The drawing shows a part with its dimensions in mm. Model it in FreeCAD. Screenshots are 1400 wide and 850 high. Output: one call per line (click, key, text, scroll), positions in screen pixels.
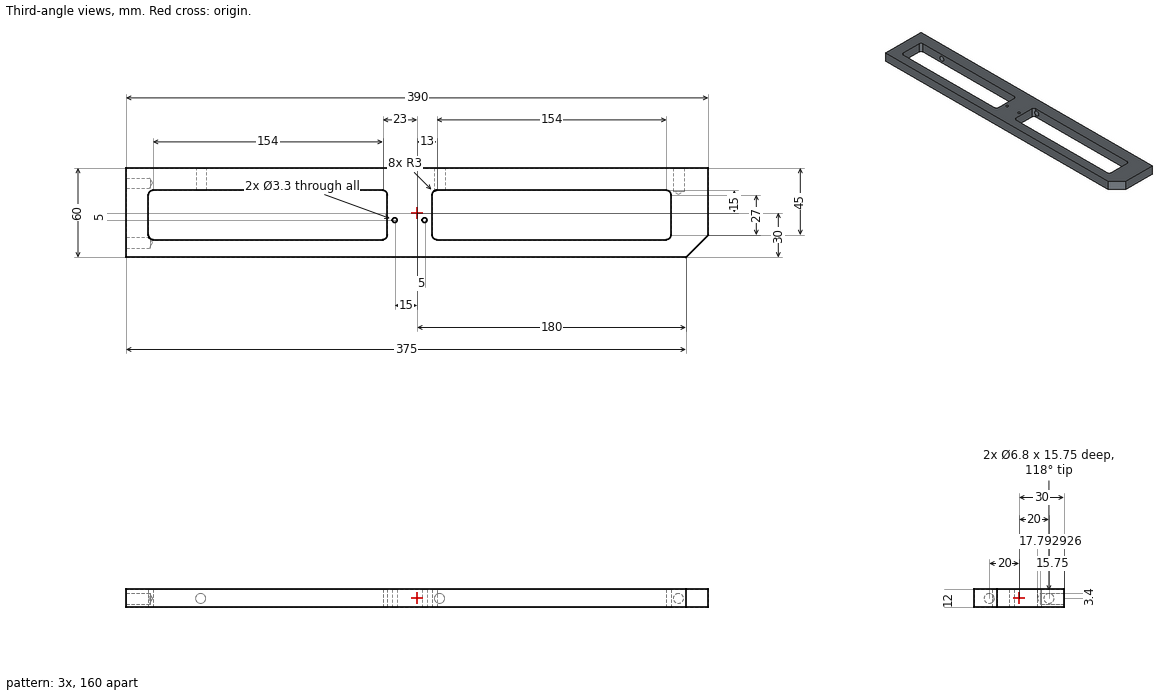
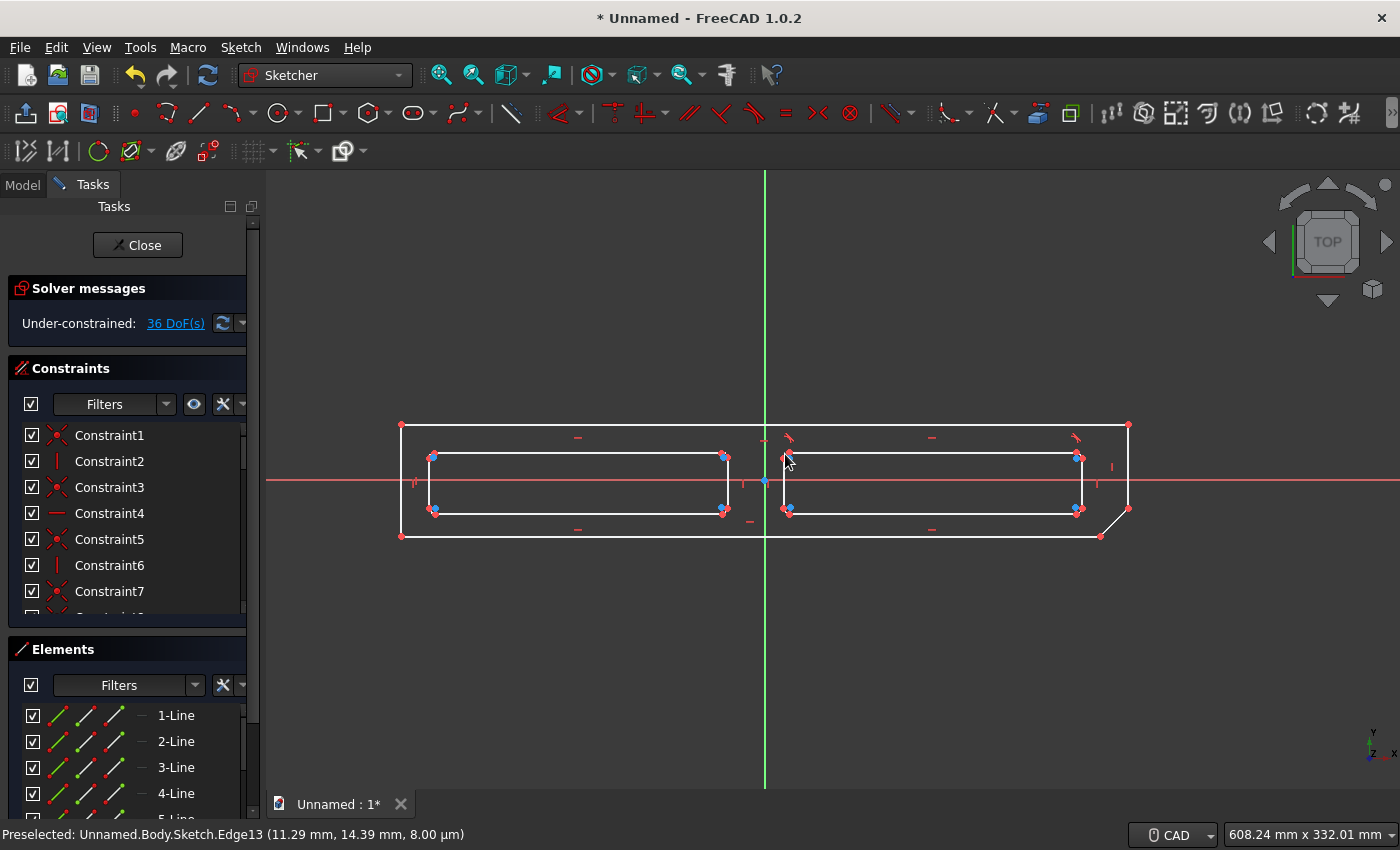
scroll(1082, 473, up, 4)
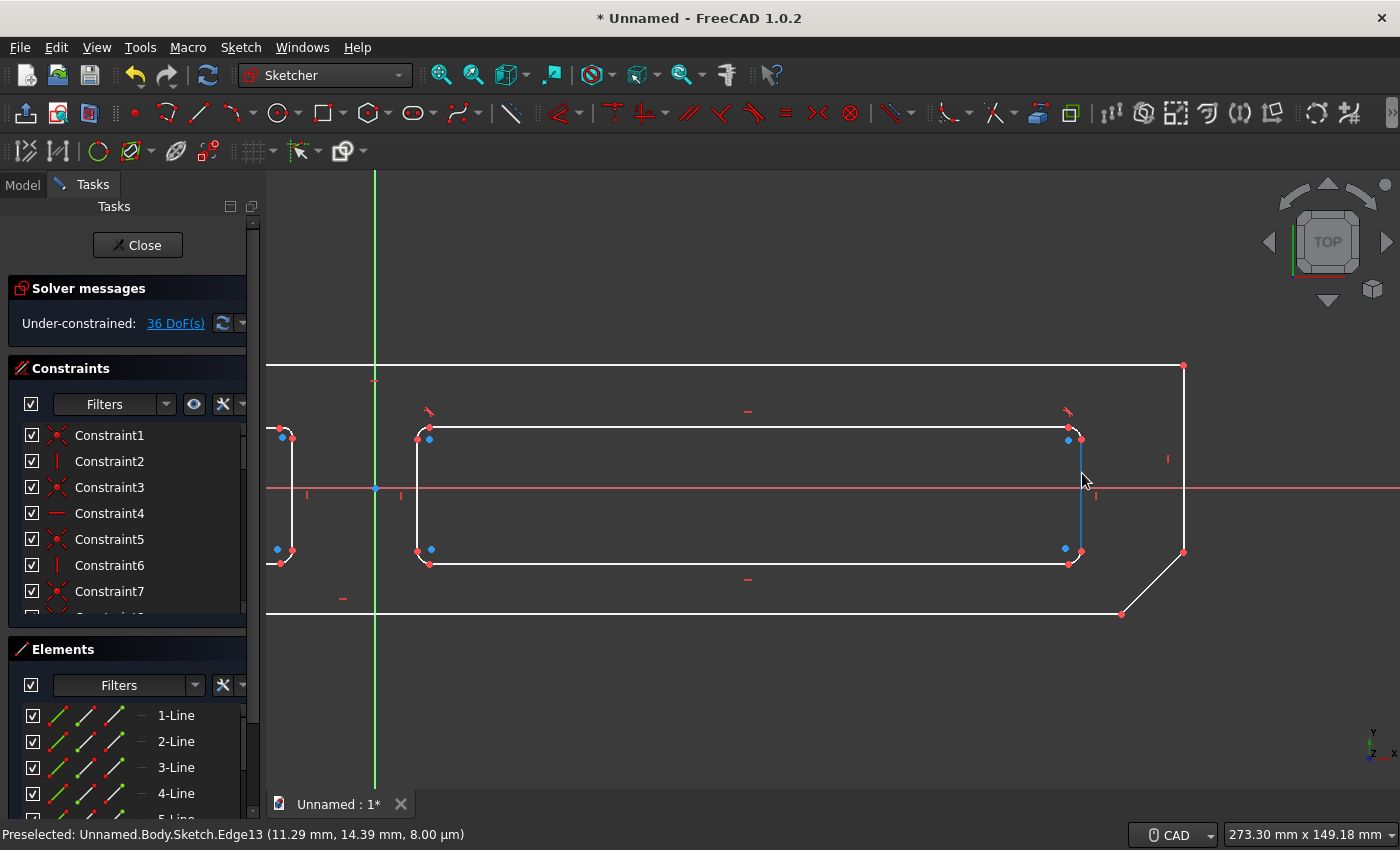
click(1081, 473)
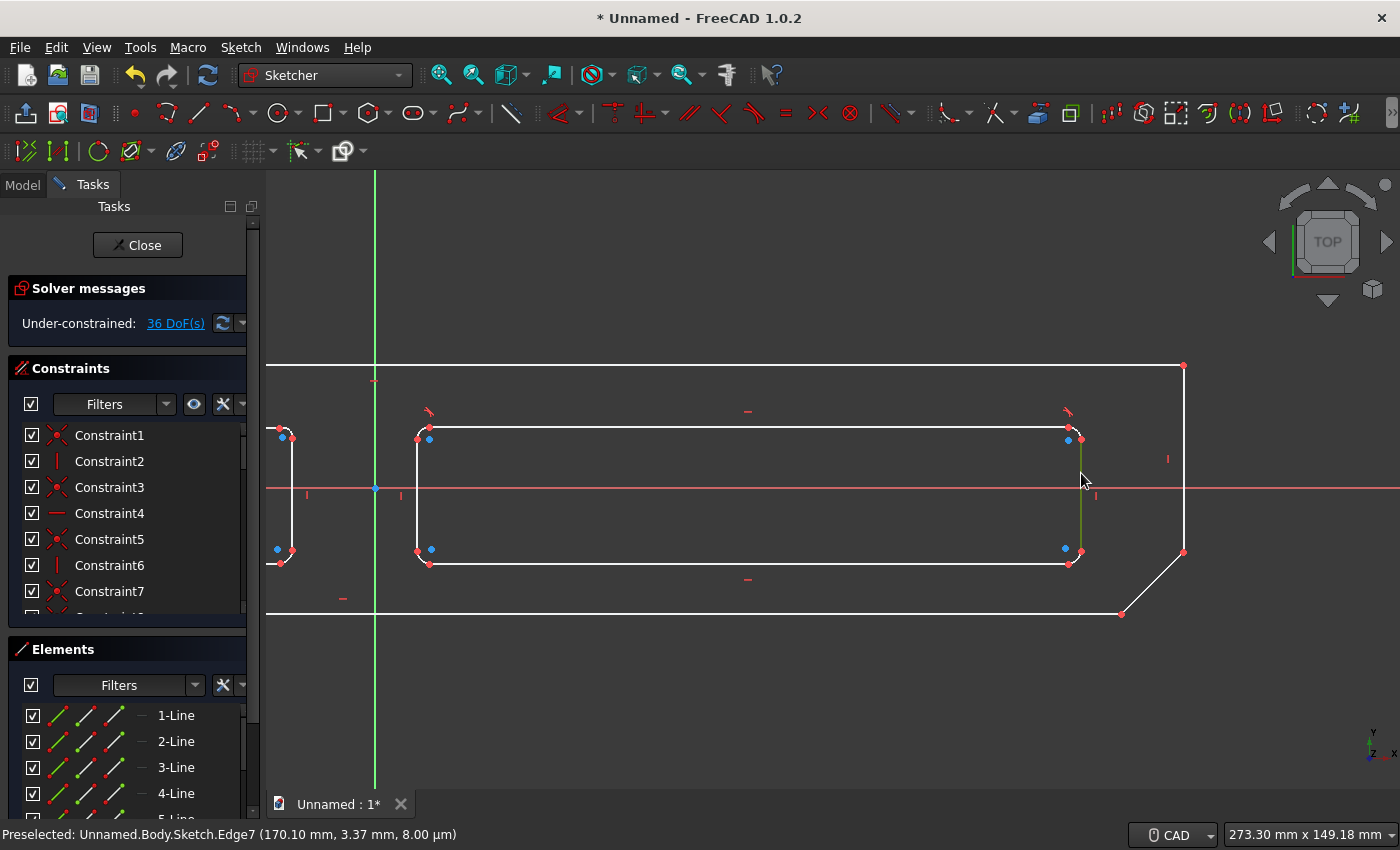
scroll(1077, 431, up, 2)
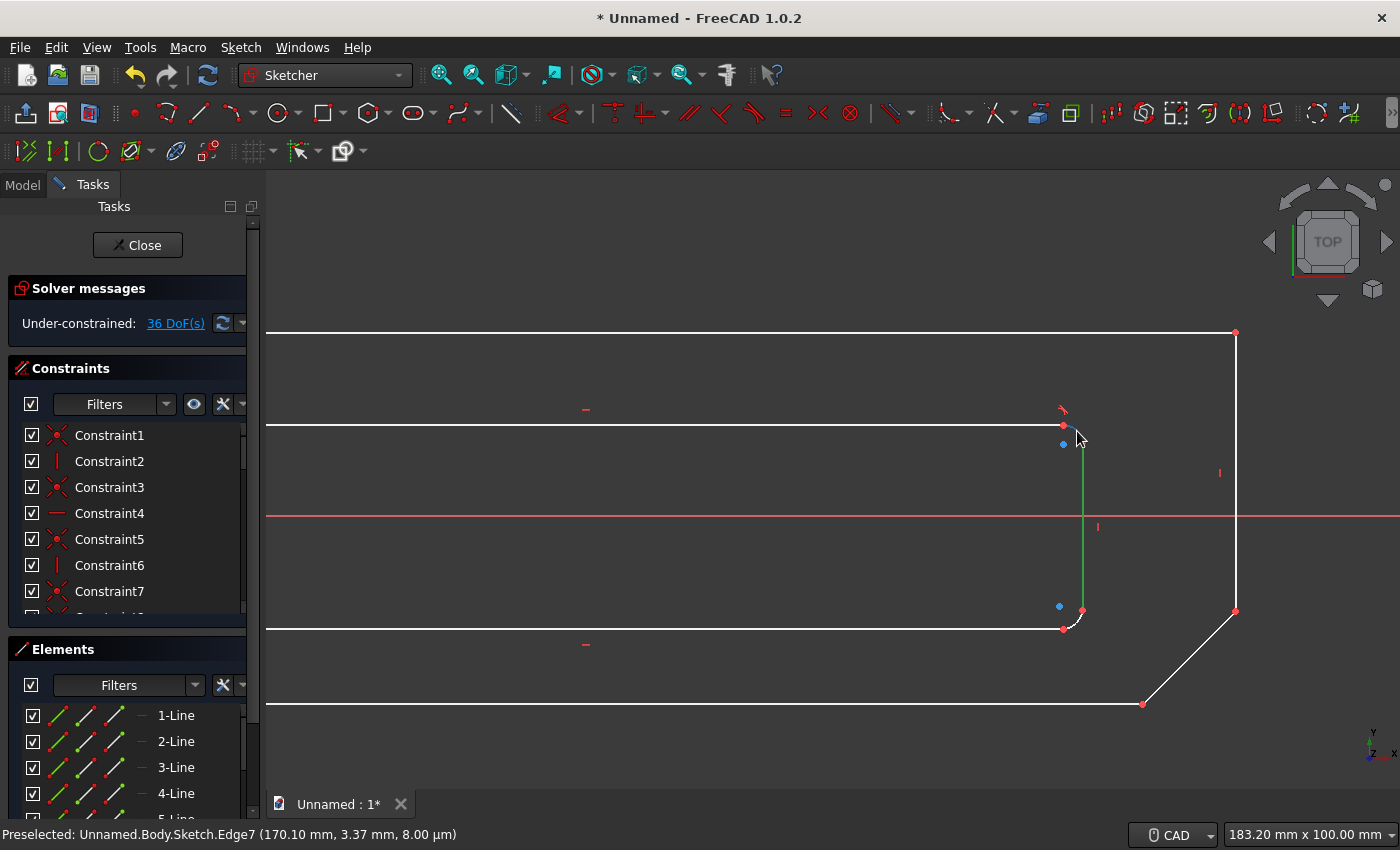
click(1077, 430)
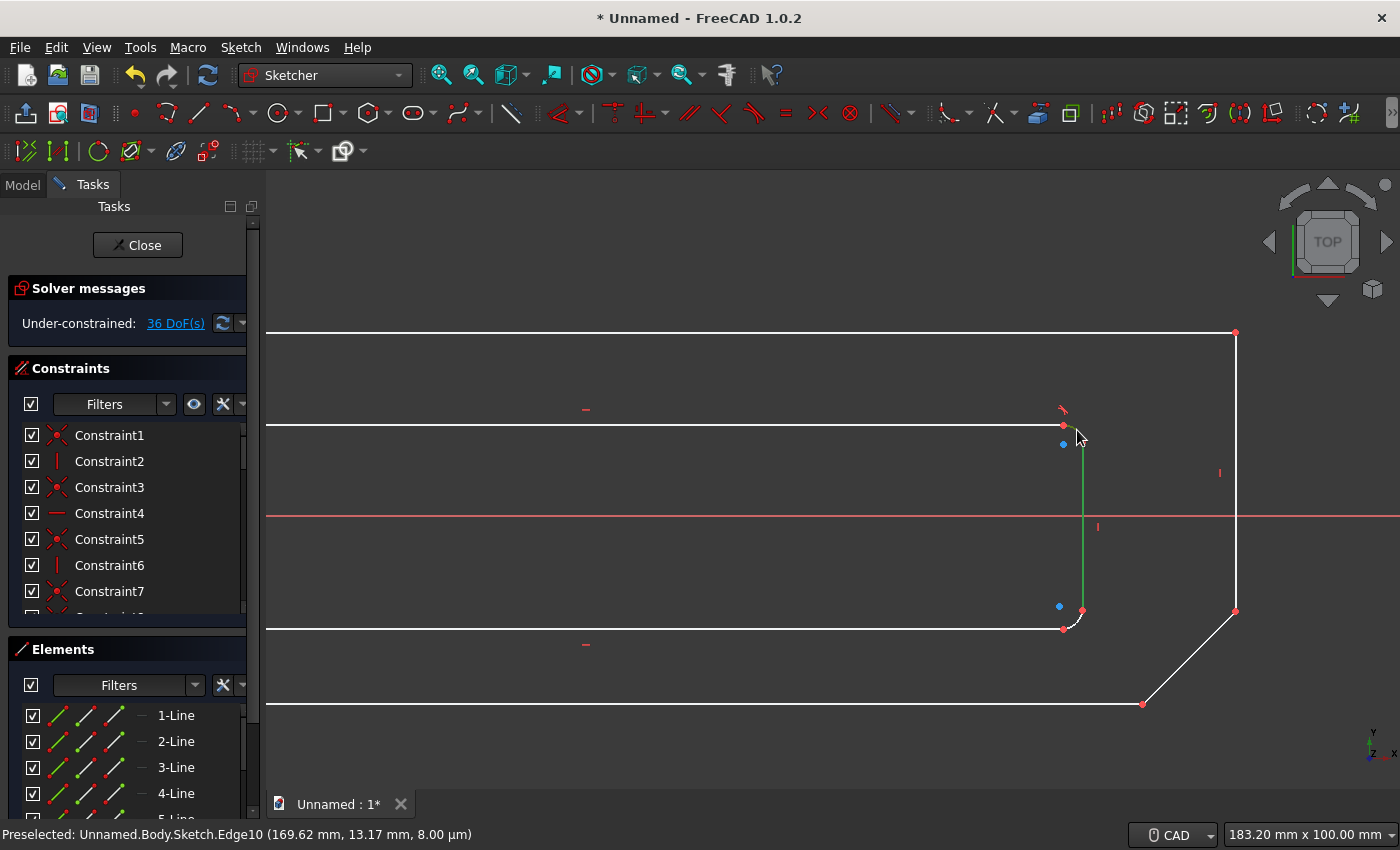
click(754, 114)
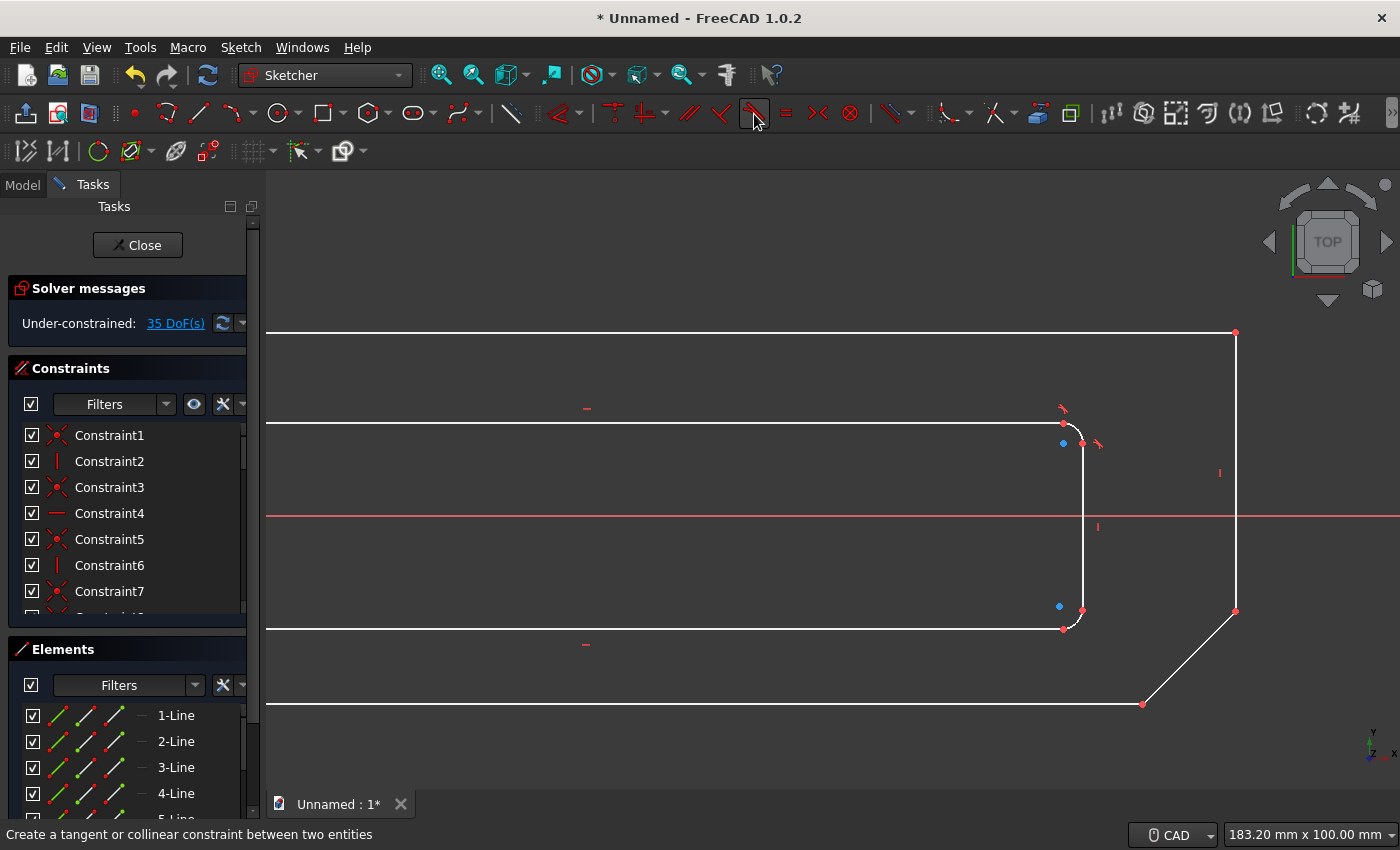
click(1083, 493)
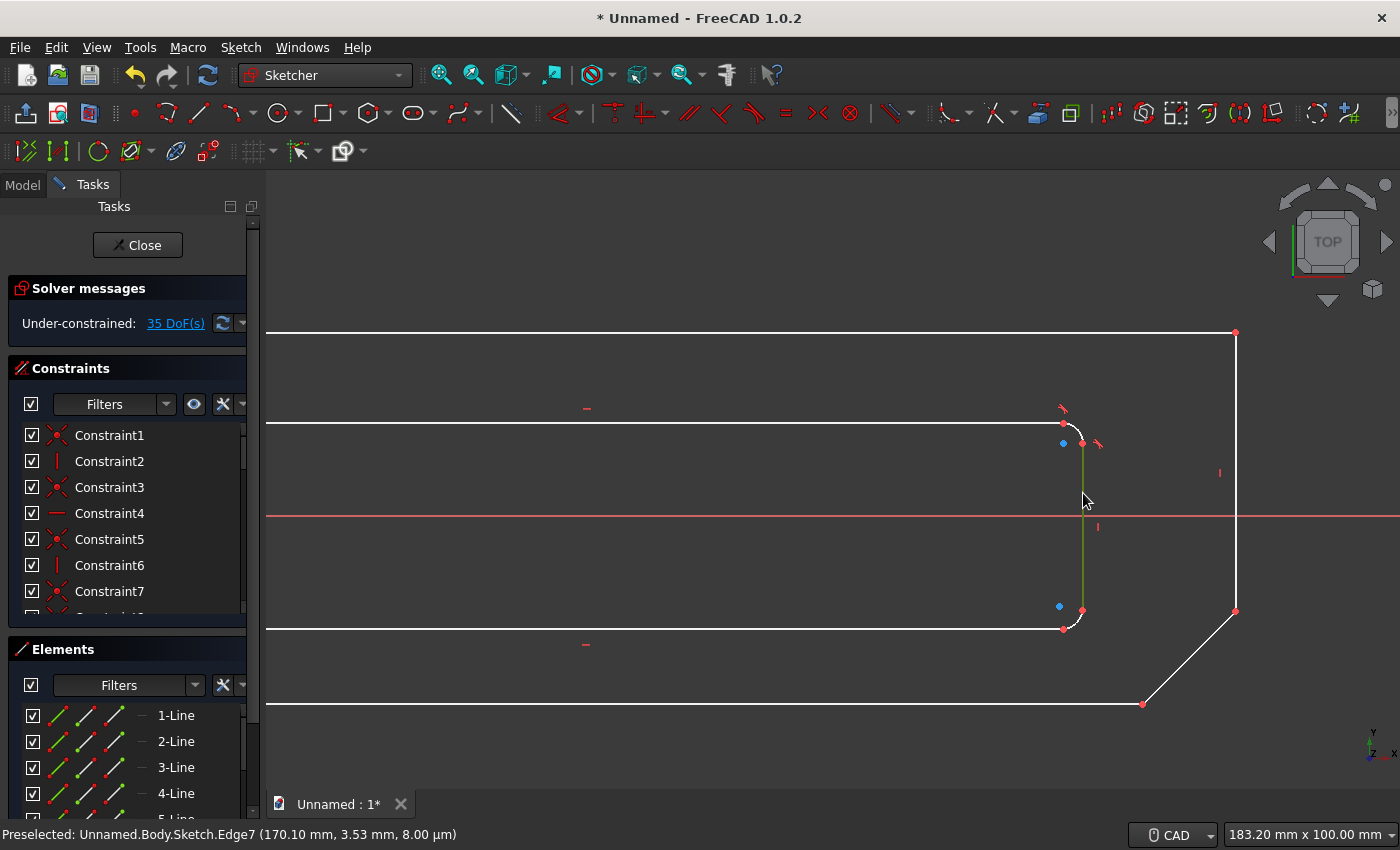
click(1076, 623)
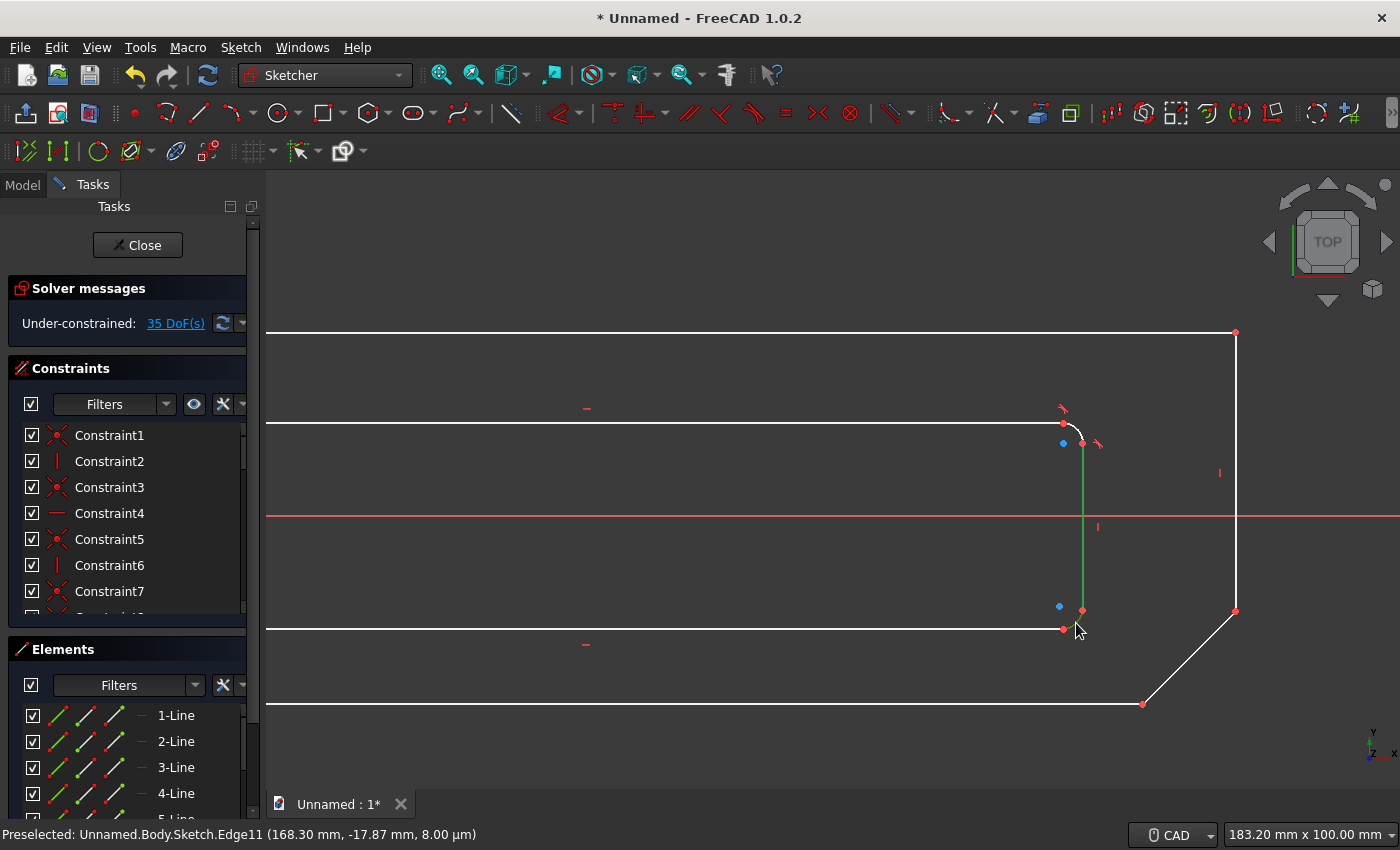
click(754, 114)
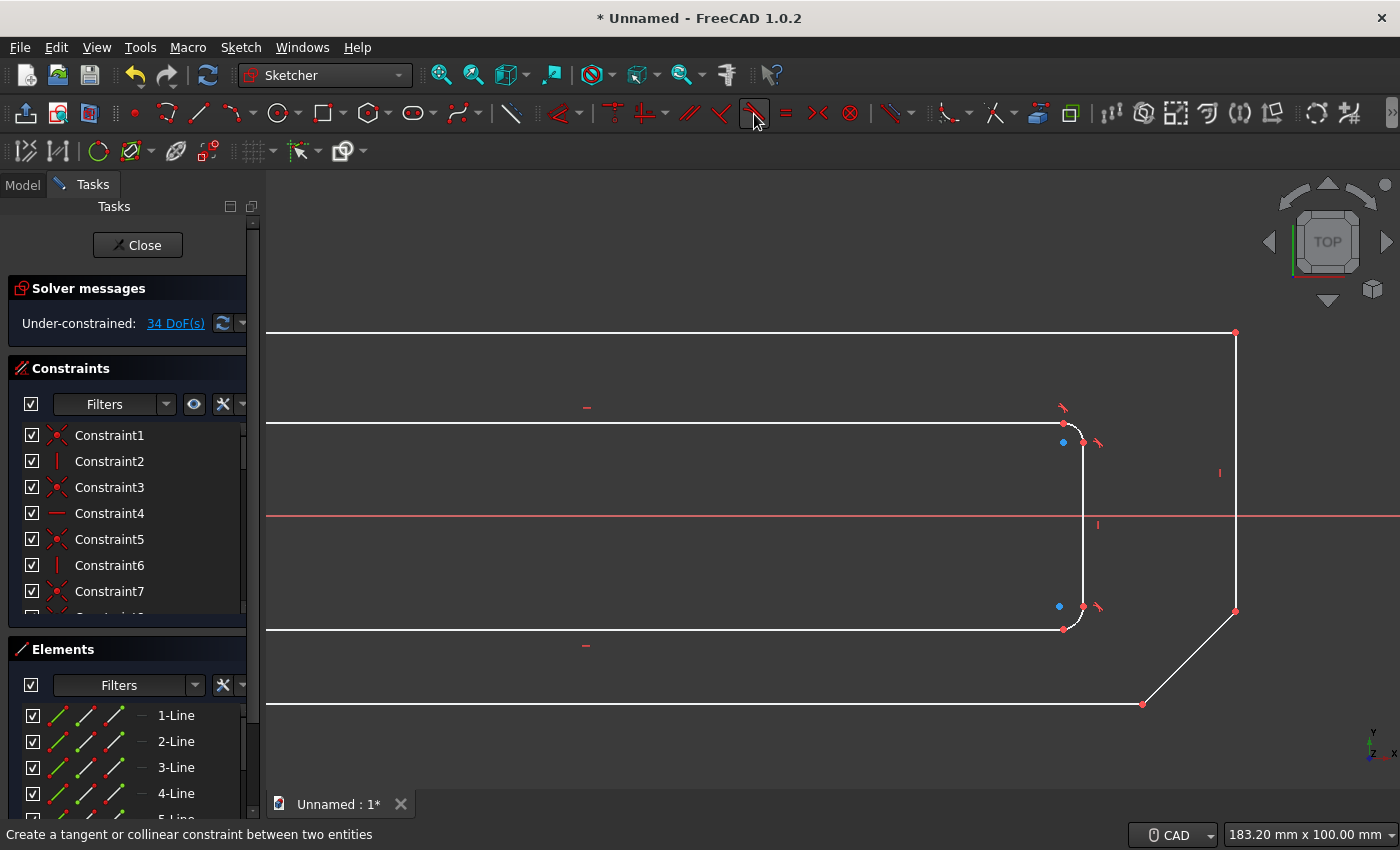
click(778, 630)